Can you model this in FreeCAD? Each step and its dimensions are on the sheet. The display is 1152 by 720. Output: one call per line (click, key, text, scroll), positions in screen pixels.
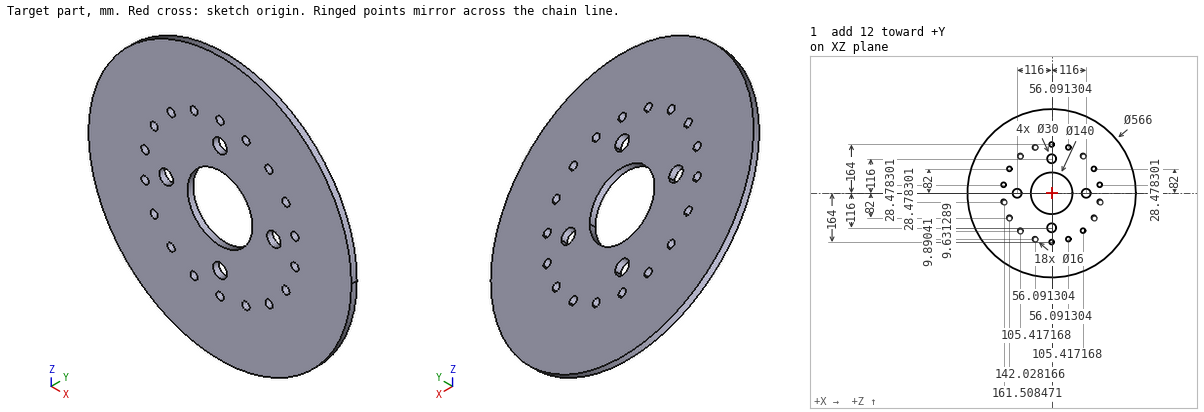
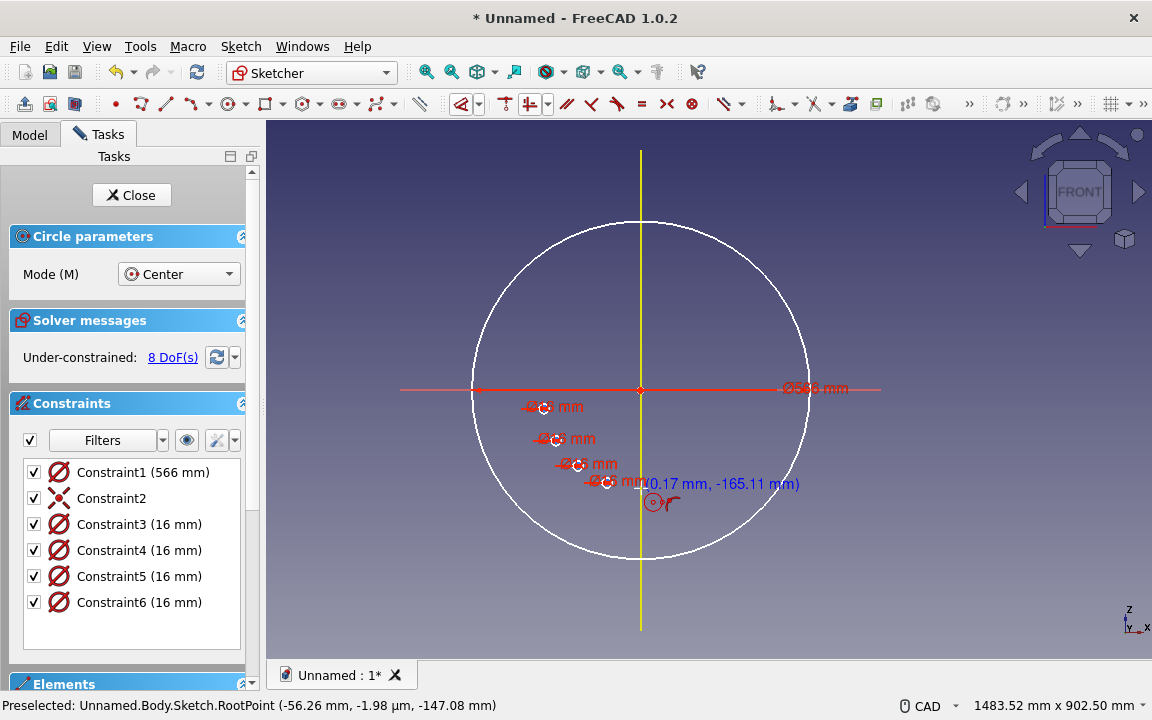
click(641, 488)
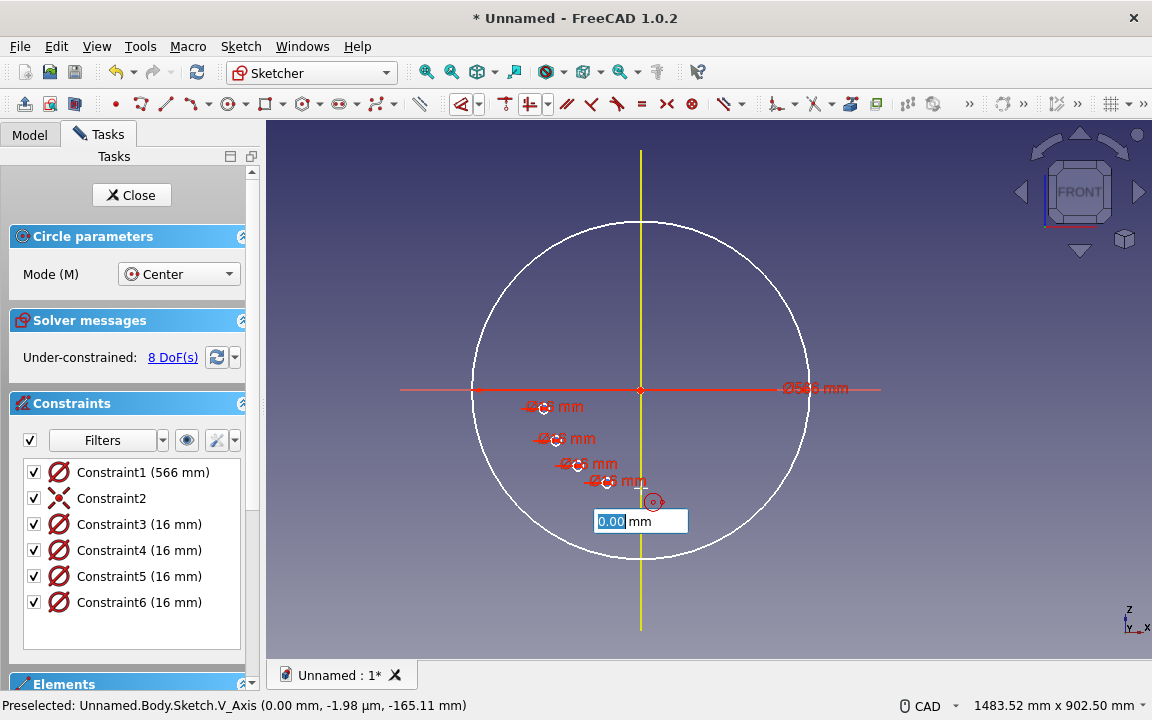
scroll(645, 487, up, 7)
move(645, 484)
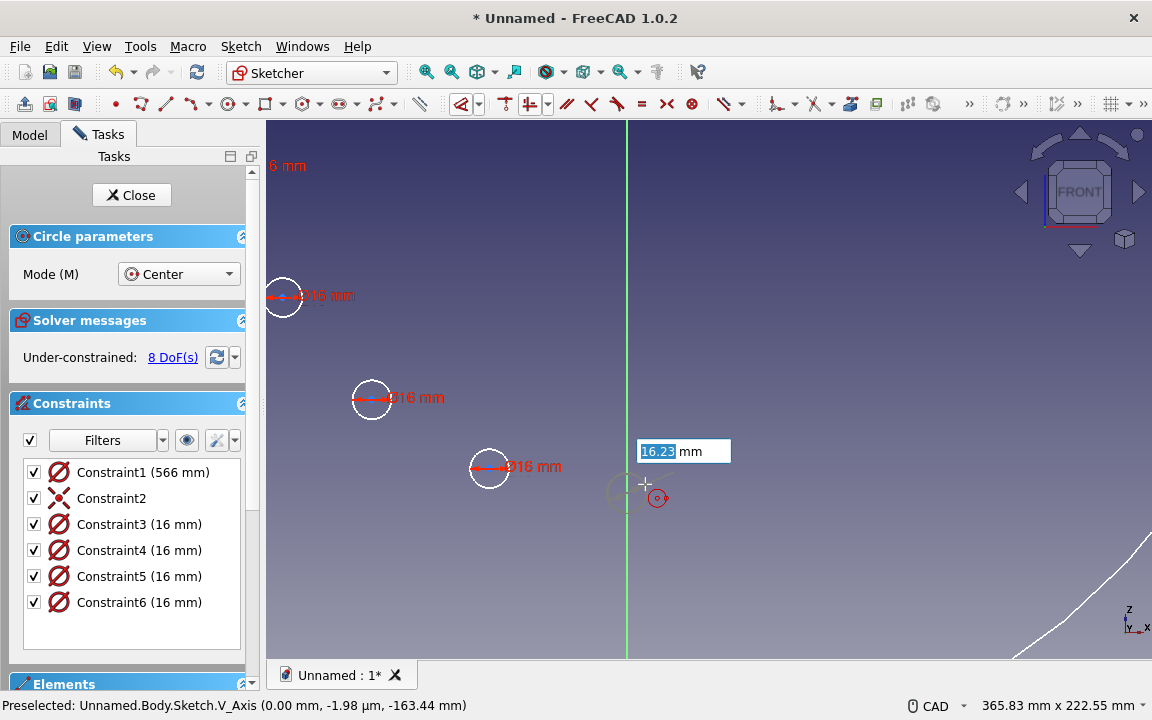
text(16)
key(Return)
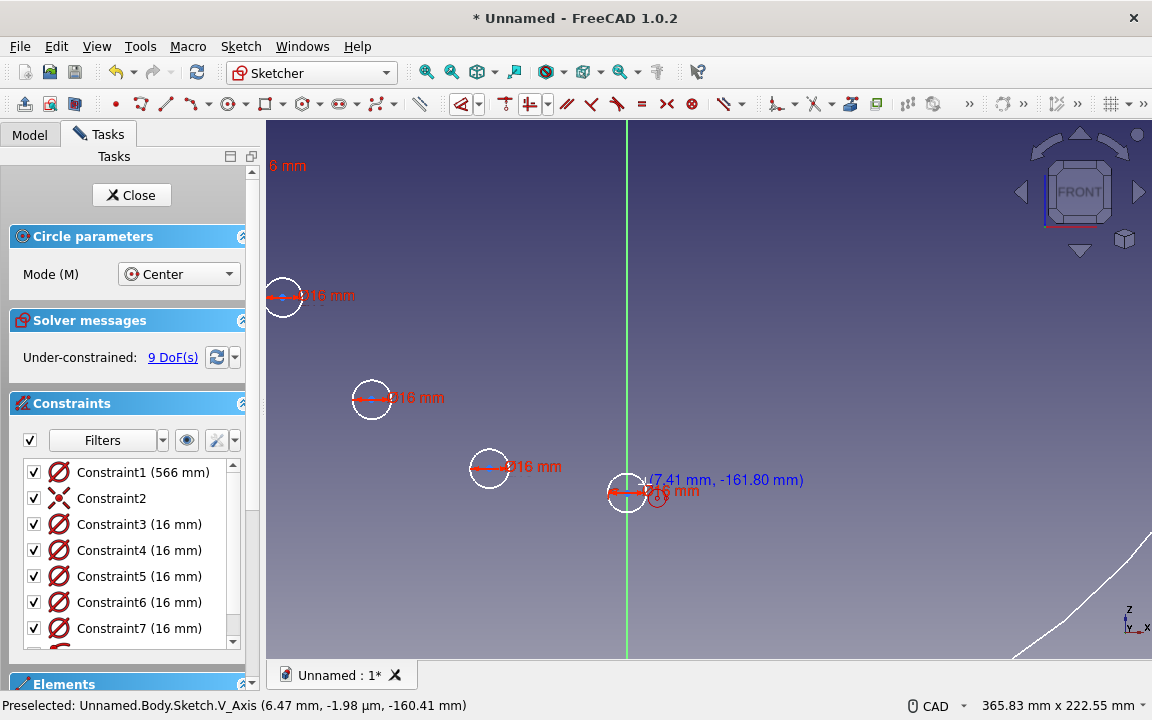
scroll(645, 486, down, 7)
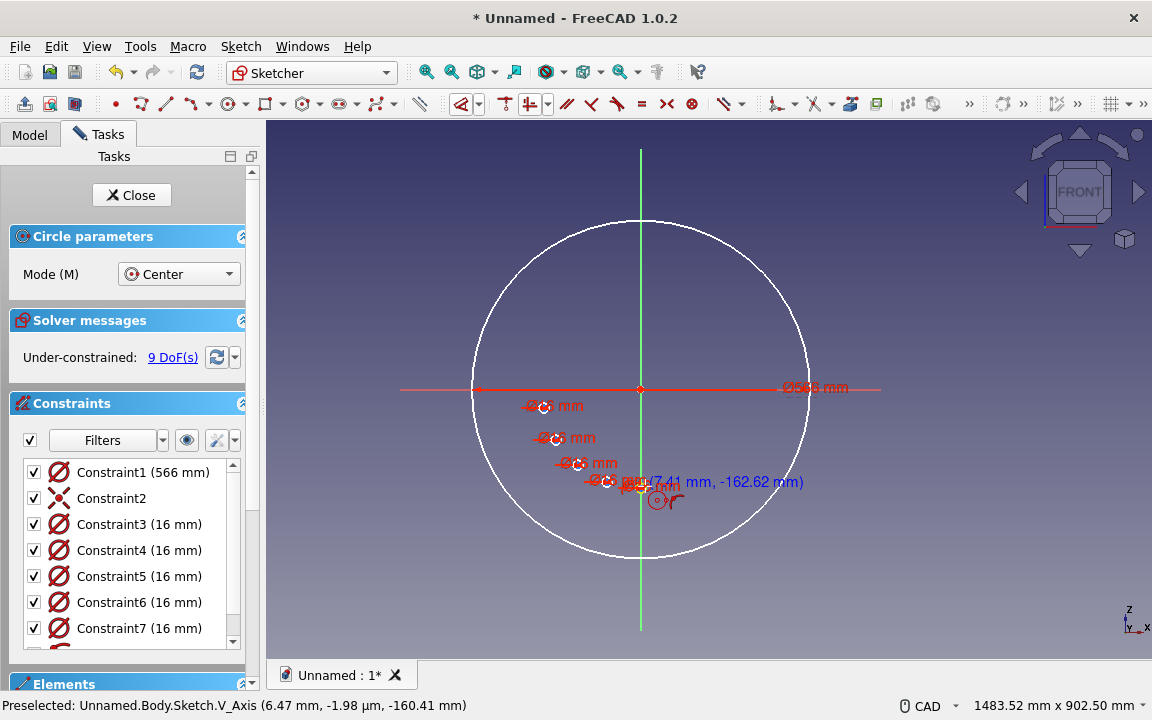
click(641, 459)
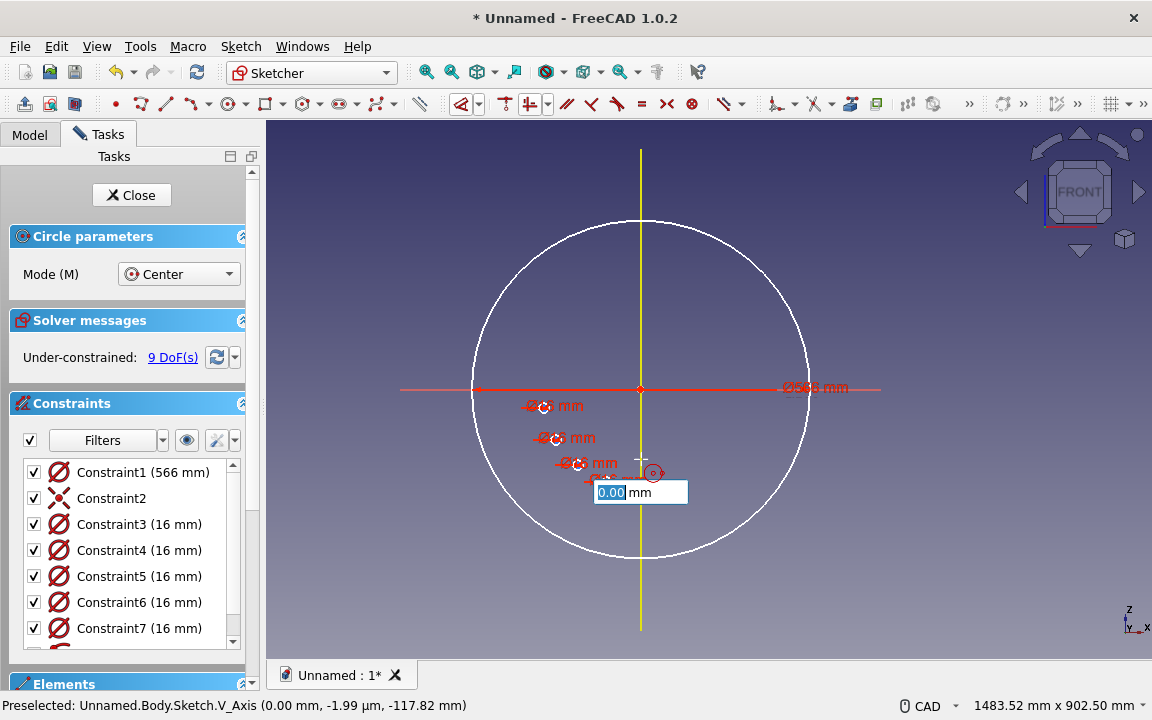
scroll(649, 456, up, 4)
move(649, 455)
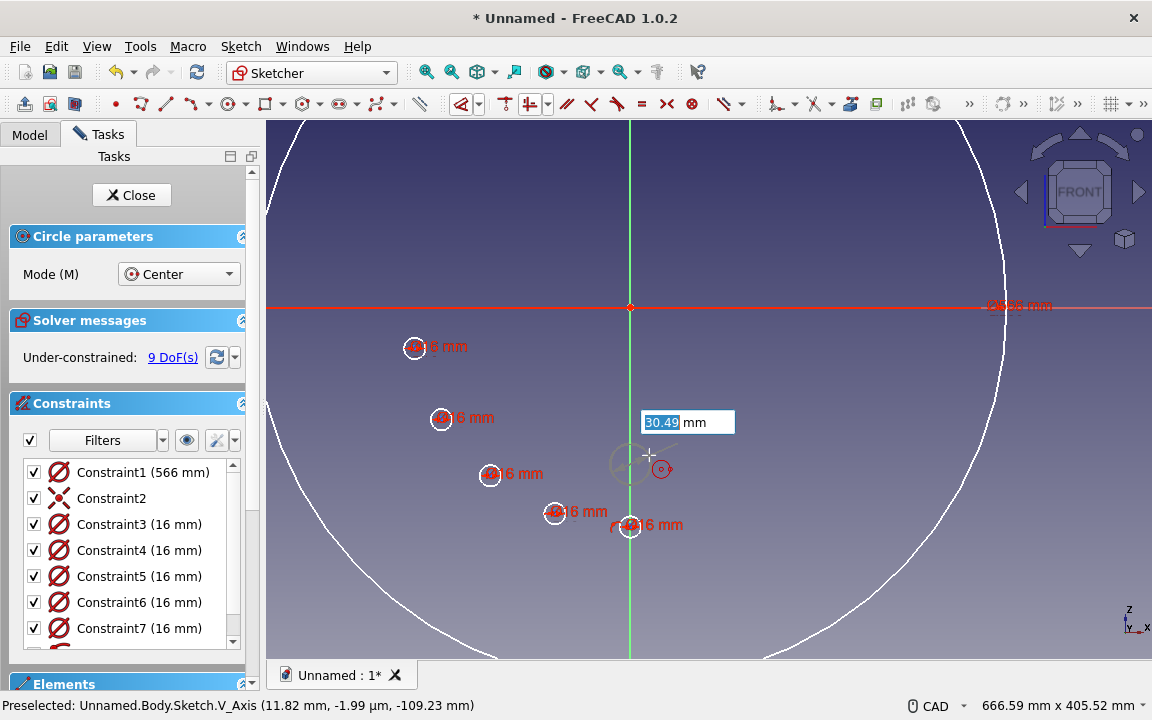
text(30)
key(Return)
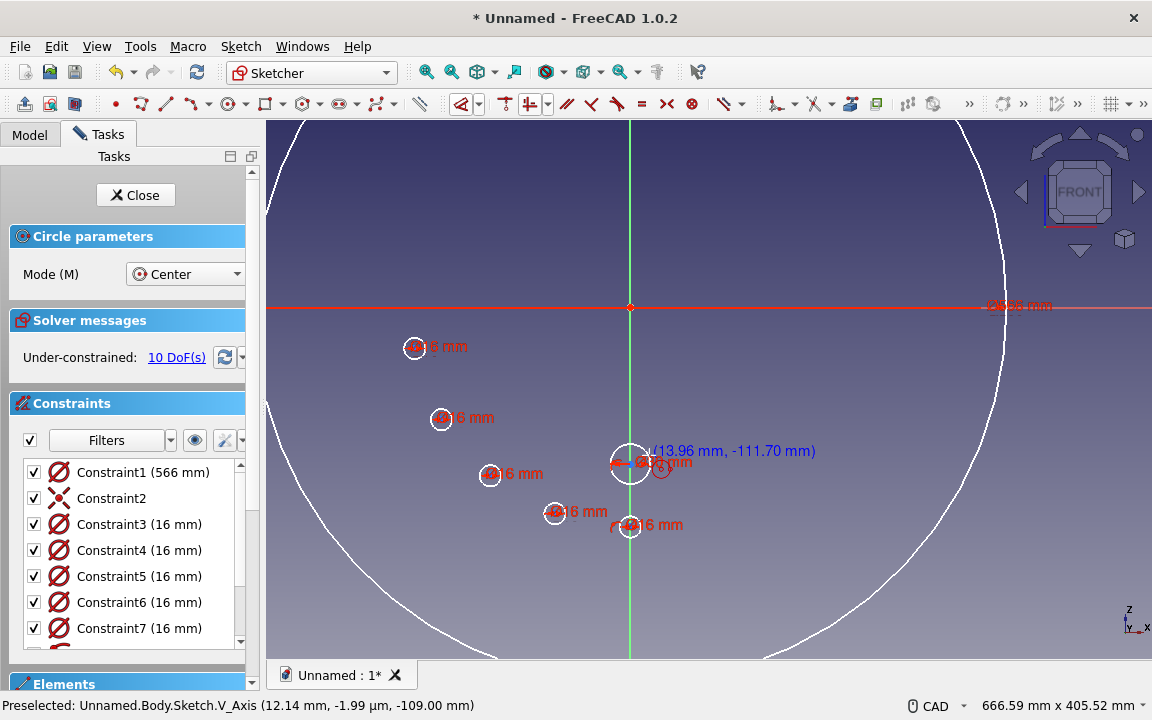
scroll(416, 270, up, 4)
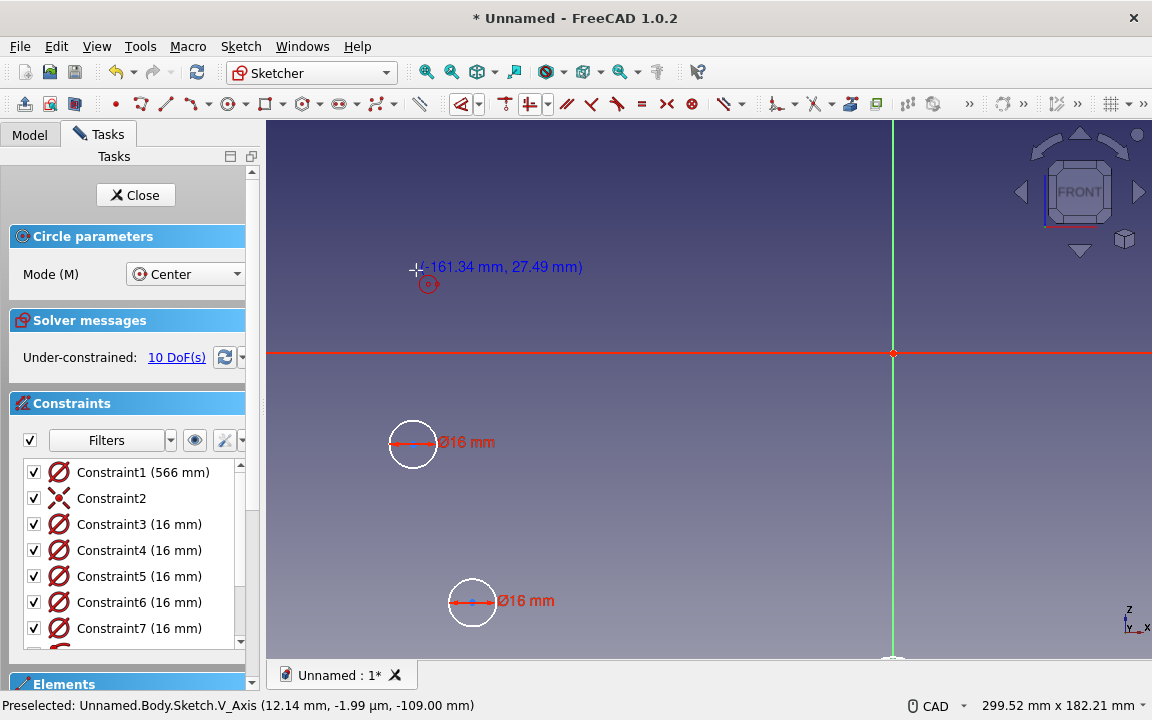
scroll(577, 399, down, 8)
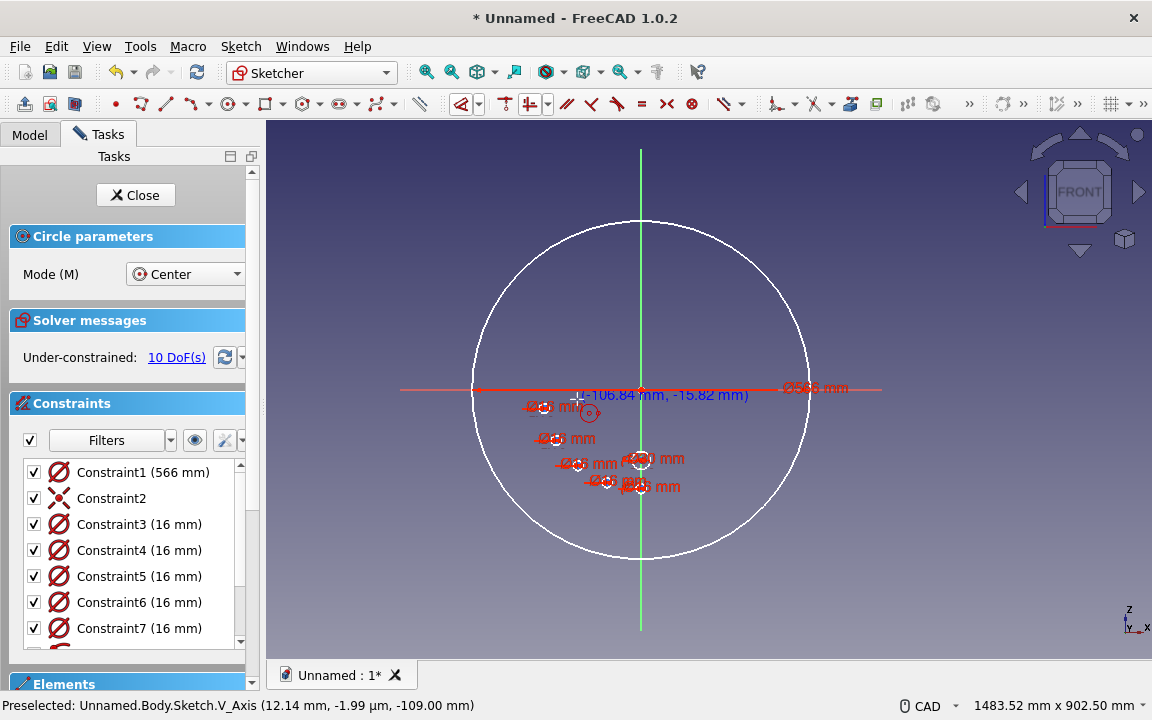
click(545, 373)
move(548, 370)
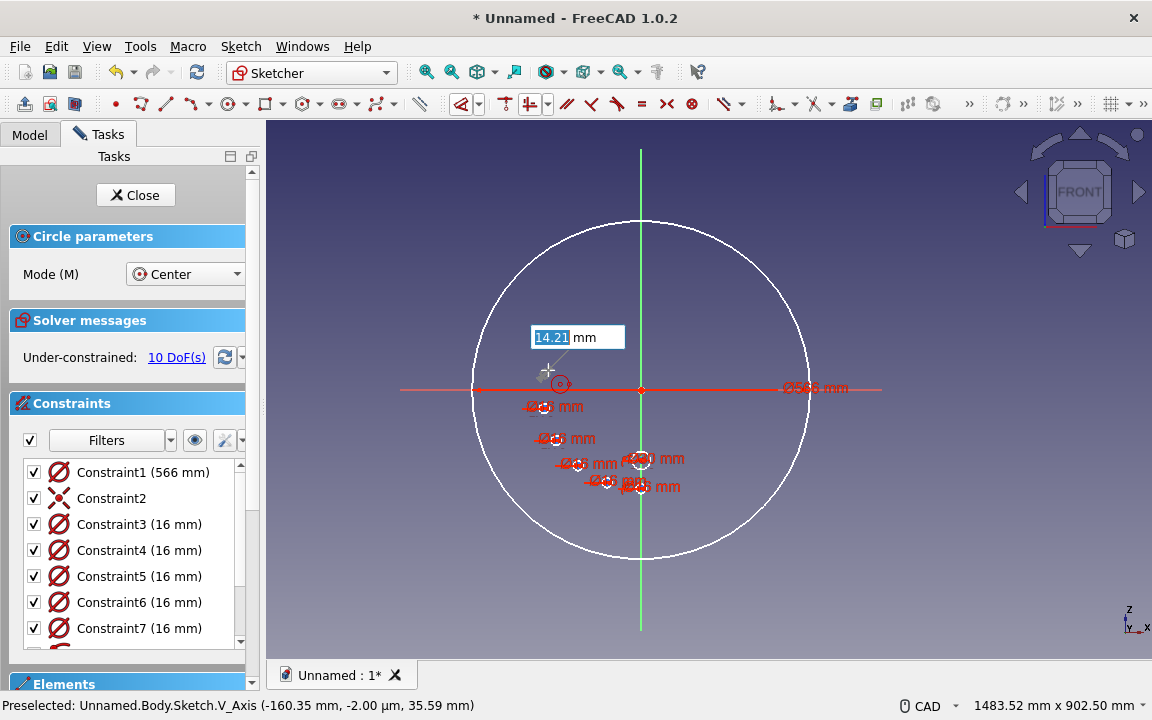
text(16)
key(Return)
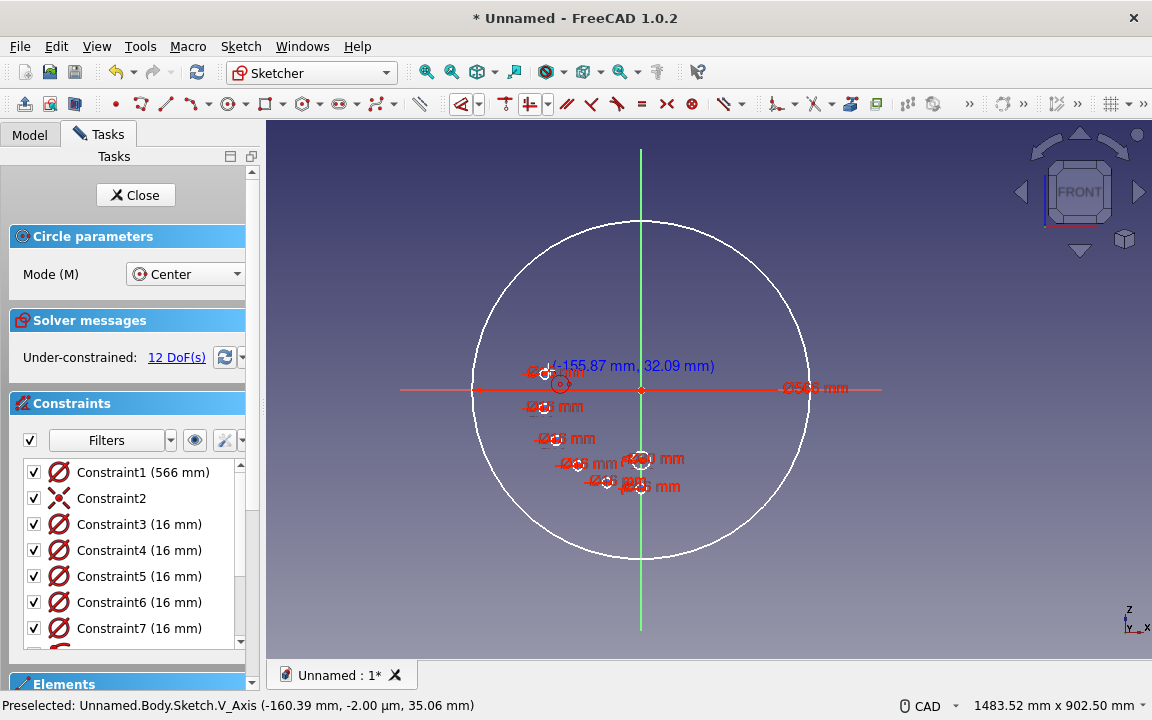
scroll(556, 341, up, 8)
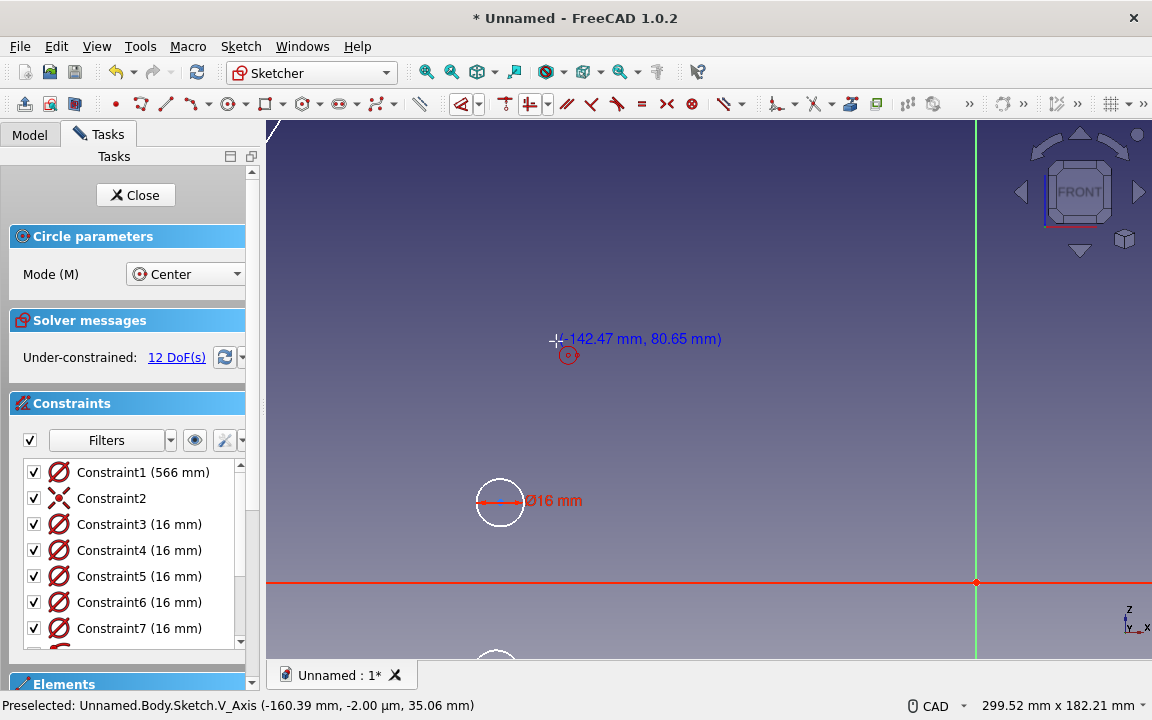
scroll(556, 341, down, 8)